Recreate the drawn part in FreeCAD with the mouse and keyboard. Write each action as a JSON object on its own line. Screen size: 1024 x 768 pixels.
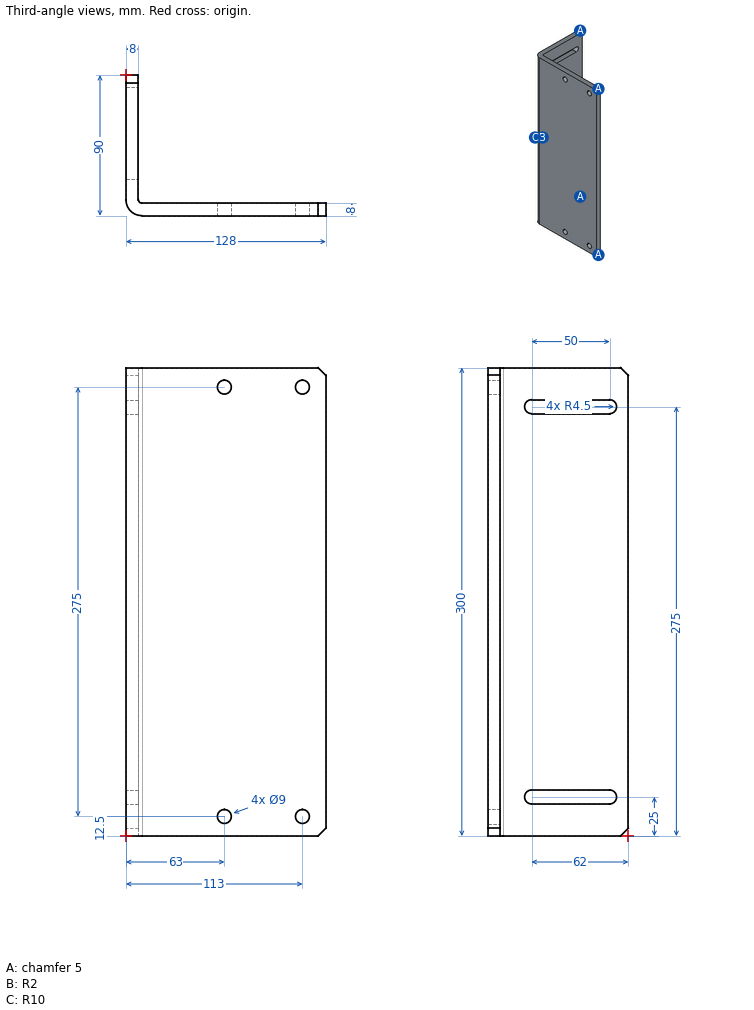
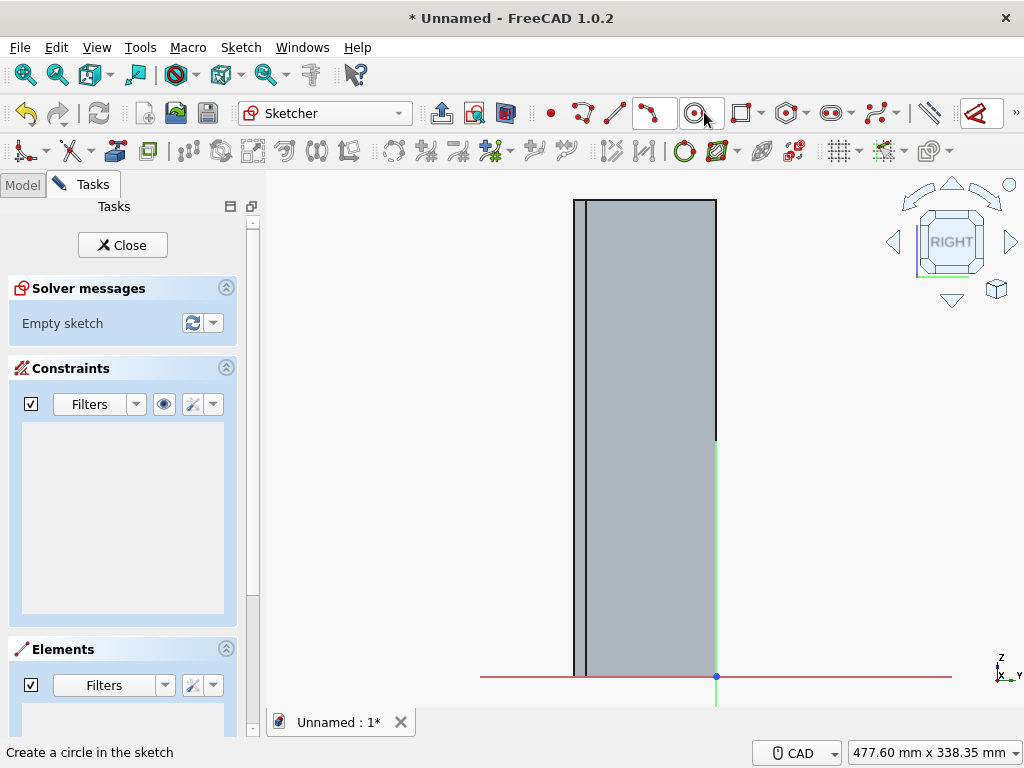
{"action": "scroll", "coordinate": [294, 365], "scroll_direction": "down", "scroll_amount": 1}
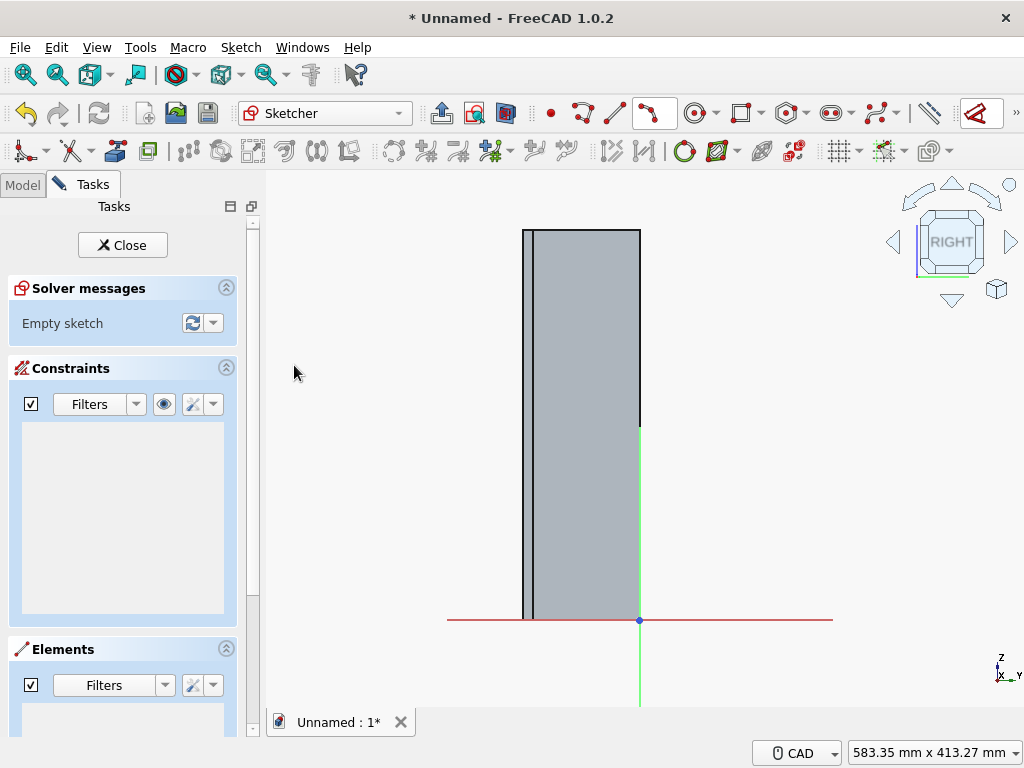
{"action": "left_click", "coordinate": [832, 114]}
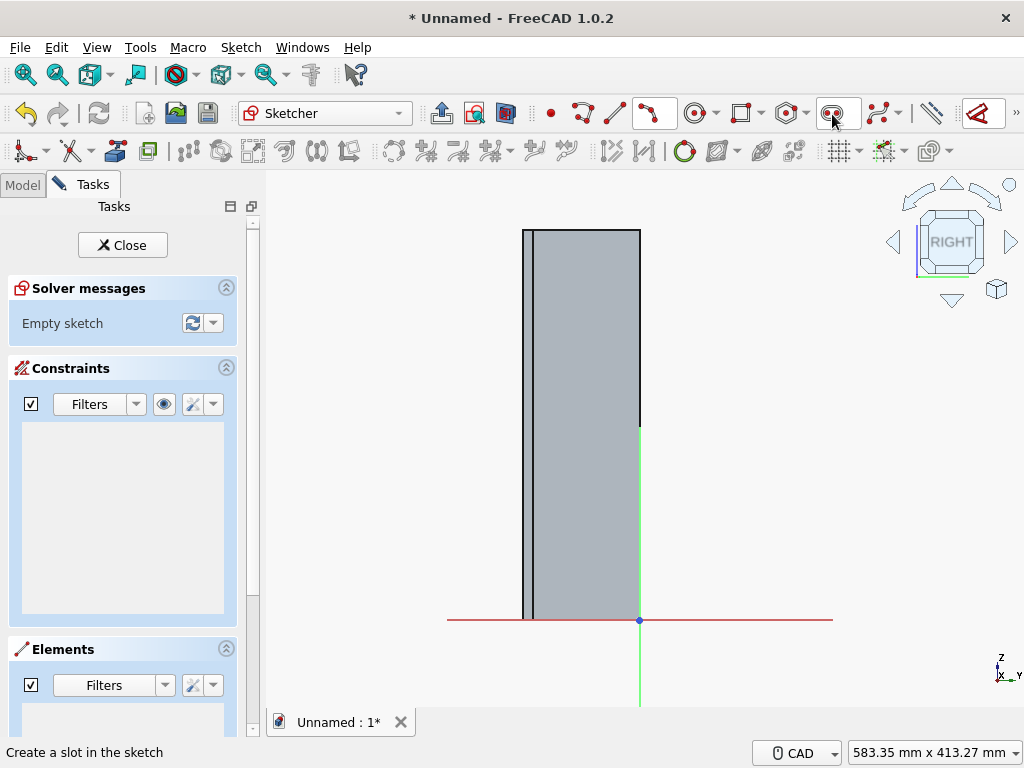
{"action": "scroll", "coordinate": [559, 263], "scroll_direction": "up", "scroll_amount": 7}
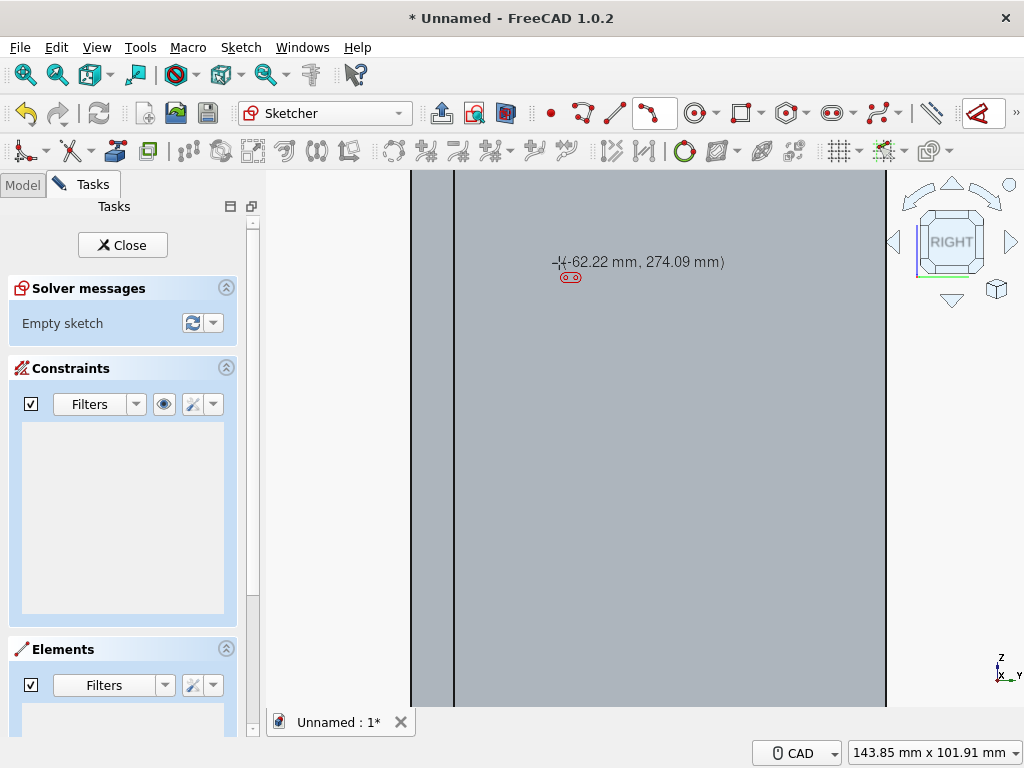
{"action": "scroll", "coordinate": [533, 263], "scroll_direction": "down", "scroll_amount": 7}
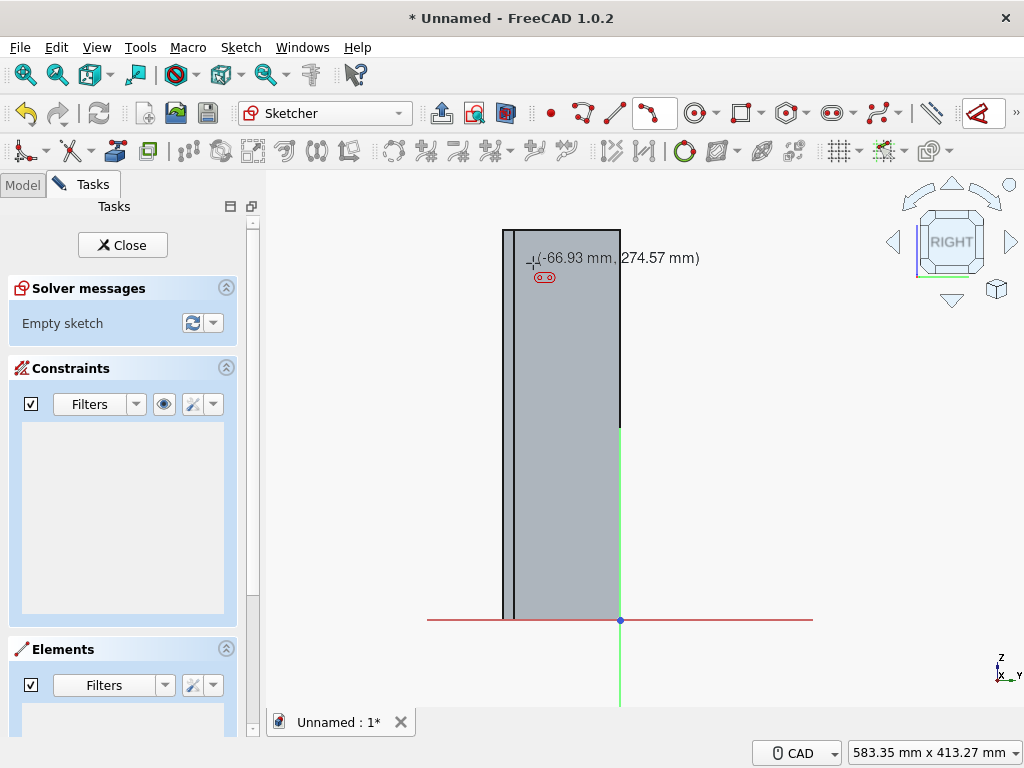
{"action": "left_click", "coordinate": [540, 263]}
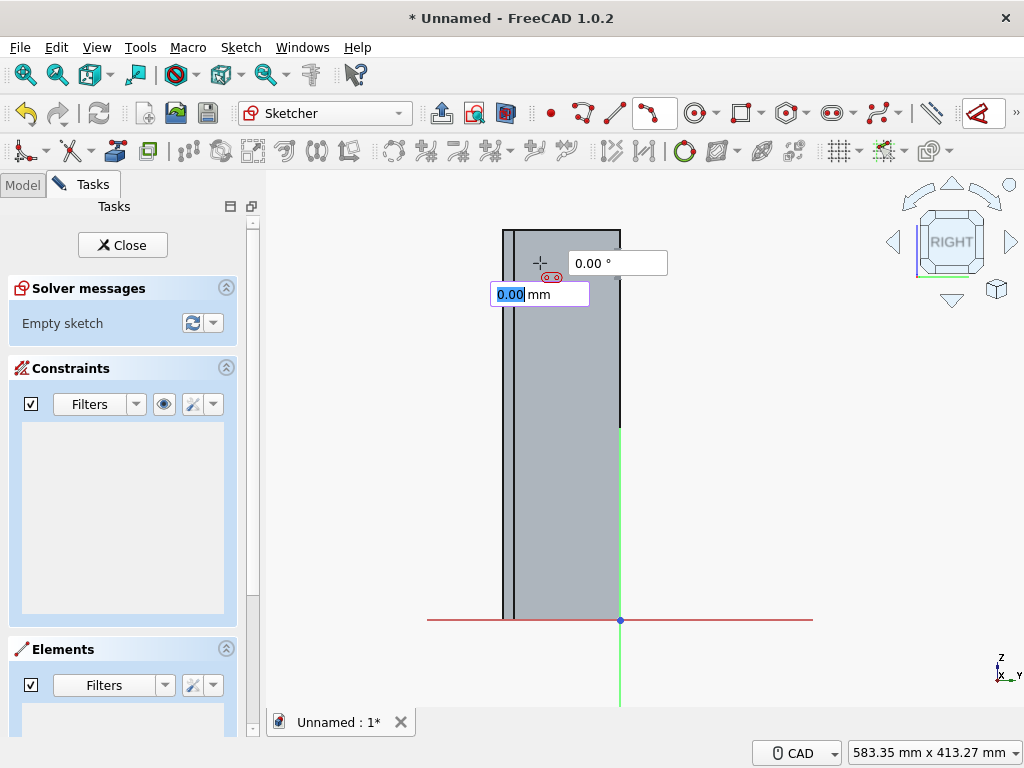
{"action": "left_click", "coordinate": [605, 263]}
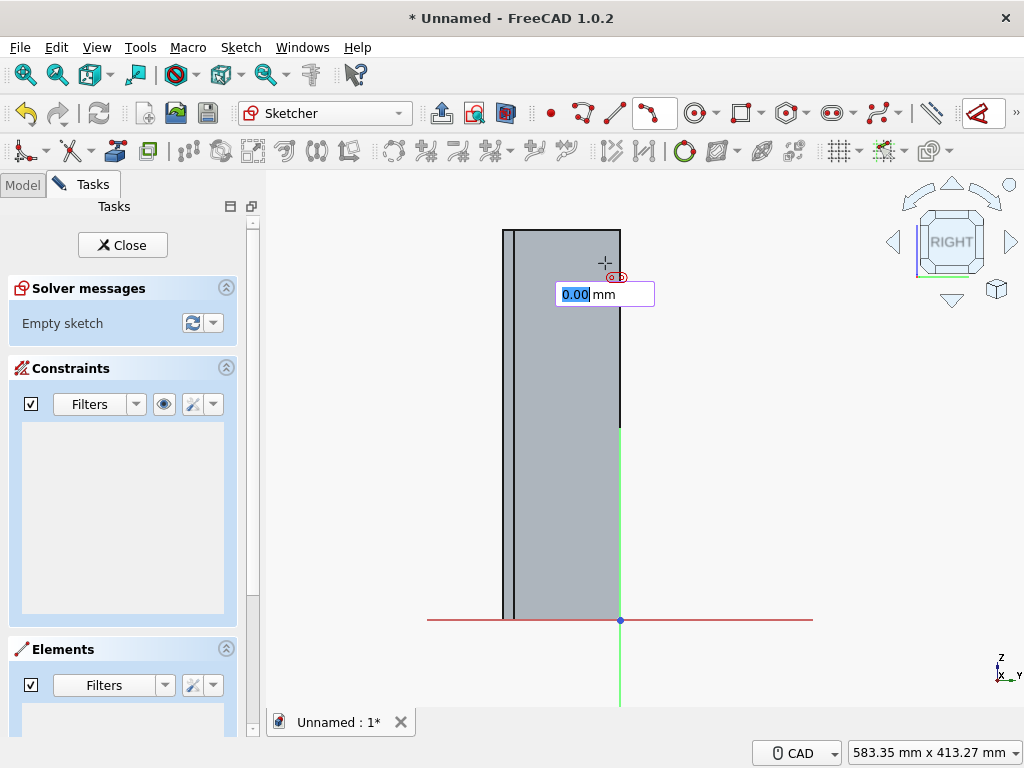
{"action": "scroll", "coordinate": [572, 269], "scroll_direction": "up", "scroll_amount": 5}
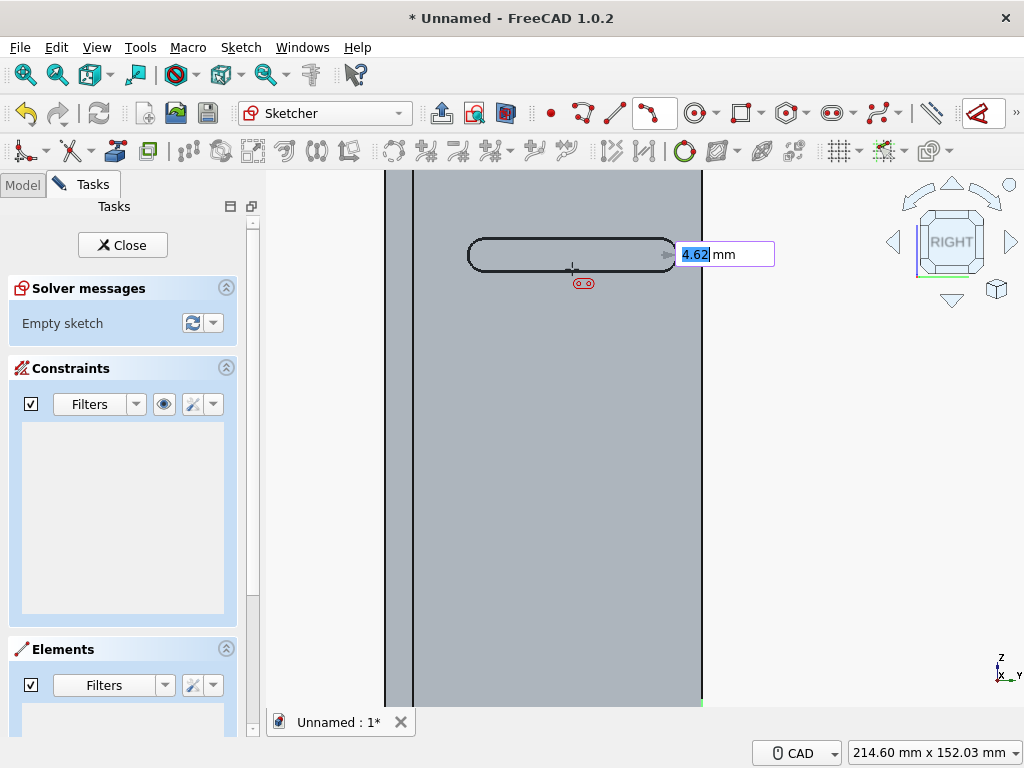
{"action": "left_click", "coordinate": [572, 268]}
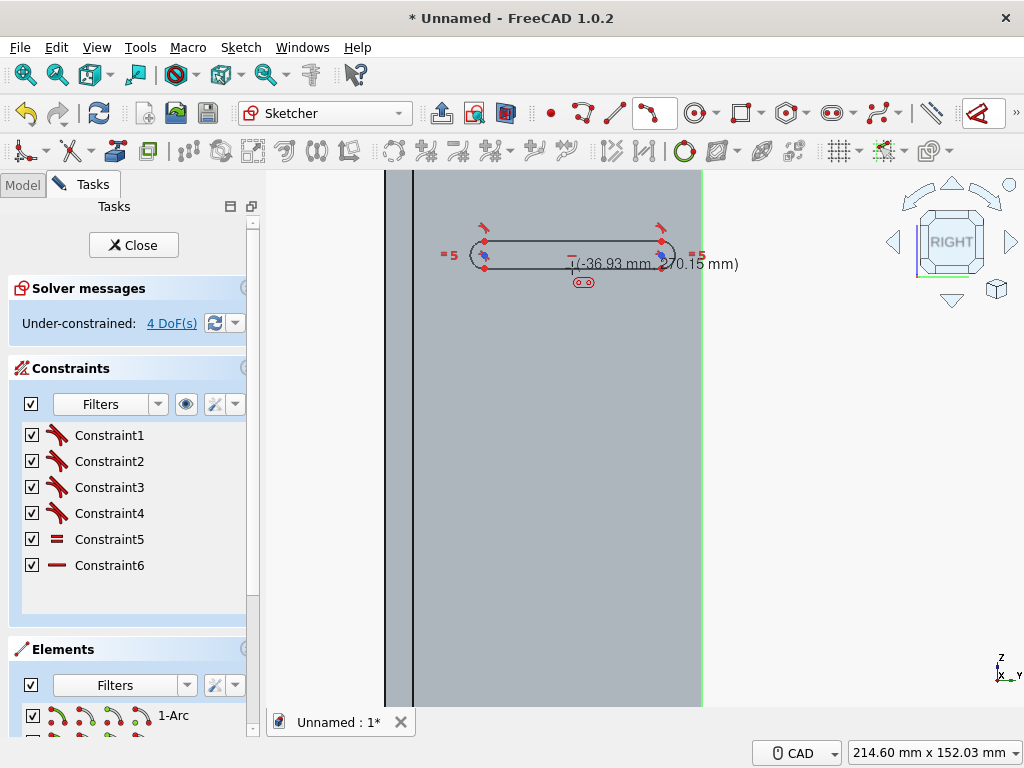
{"action": "scroll", "coordinate": [572, 269], "scroll_direction": "down", "scroll_amount": 5}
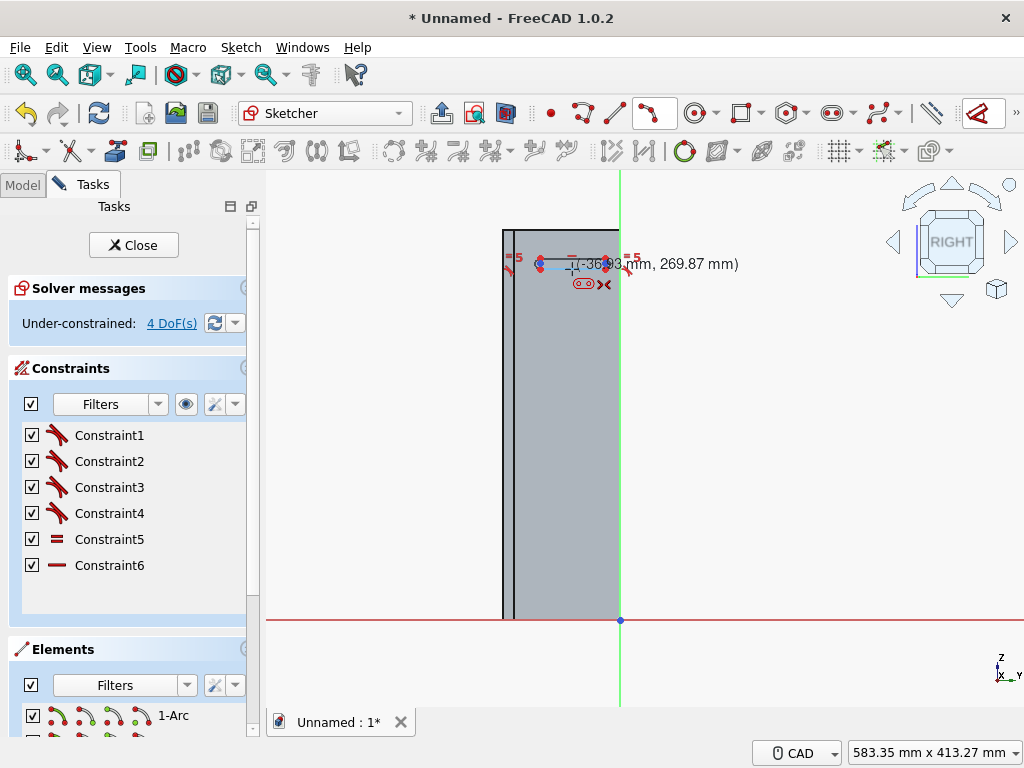
{"action": "scroll", "coordinate": [540, 588], "scroll_direction": "up", "scroll_amount": 7}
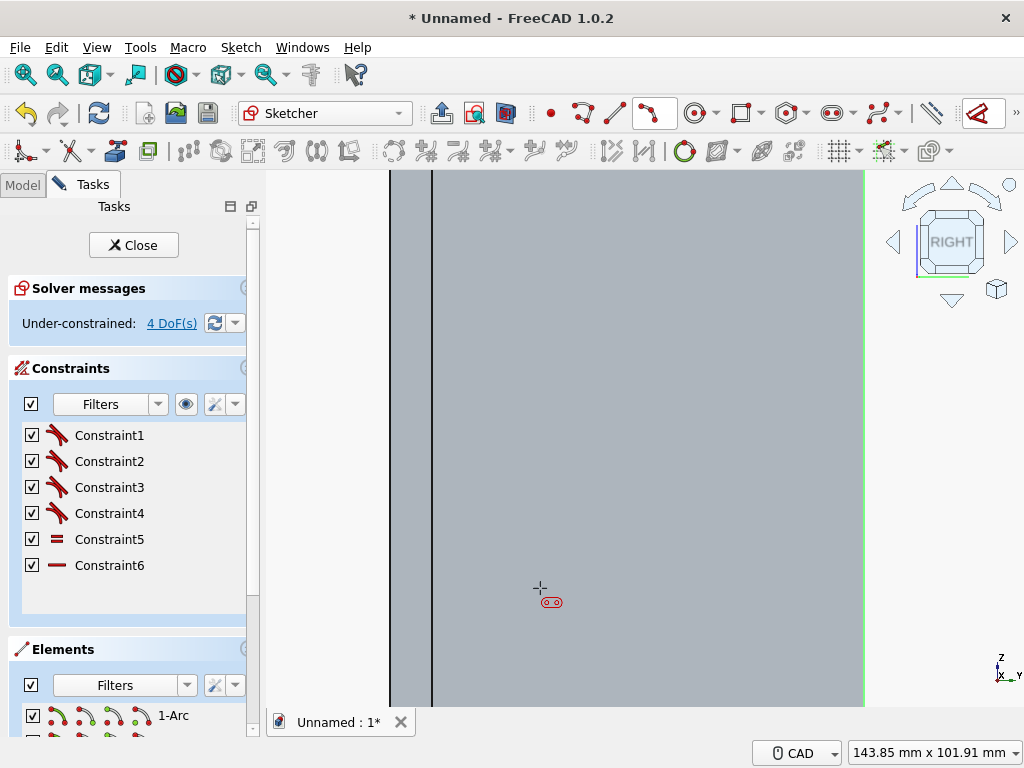
{"action": "scroll", "coordinate": [540, 589], "scroll_direction": "down", "scroll_amount": 7}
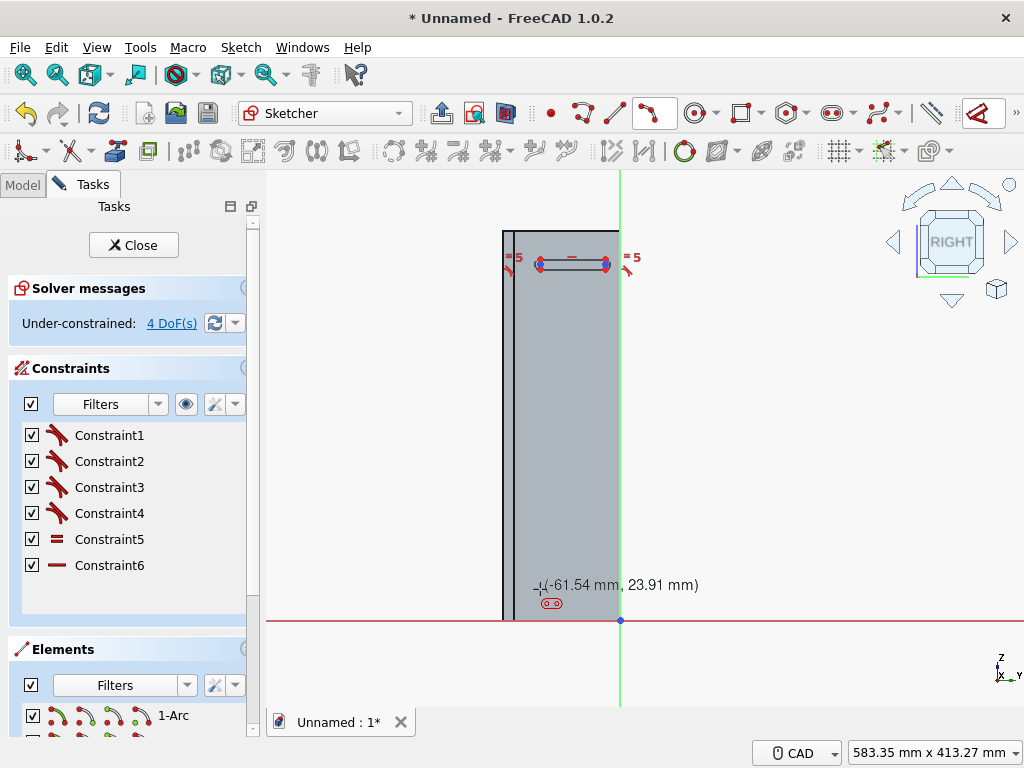
{"action": "left_click", "coordinate": [540, 588]}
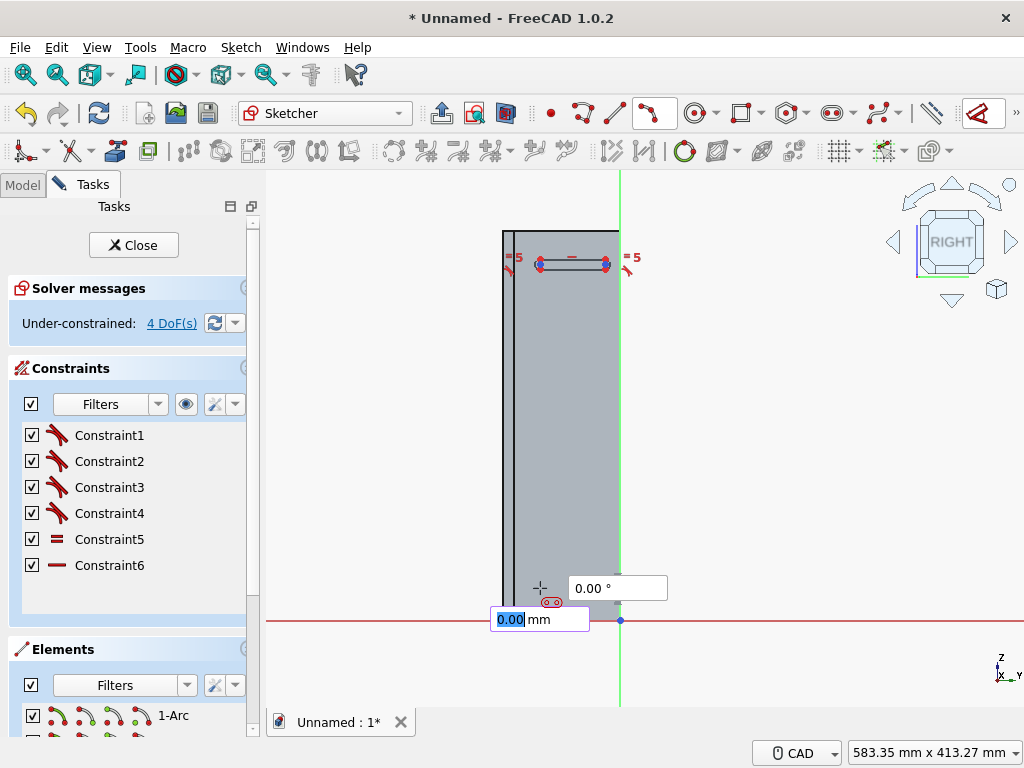
{"action": "left_click", "coordinate": [605, 588]}